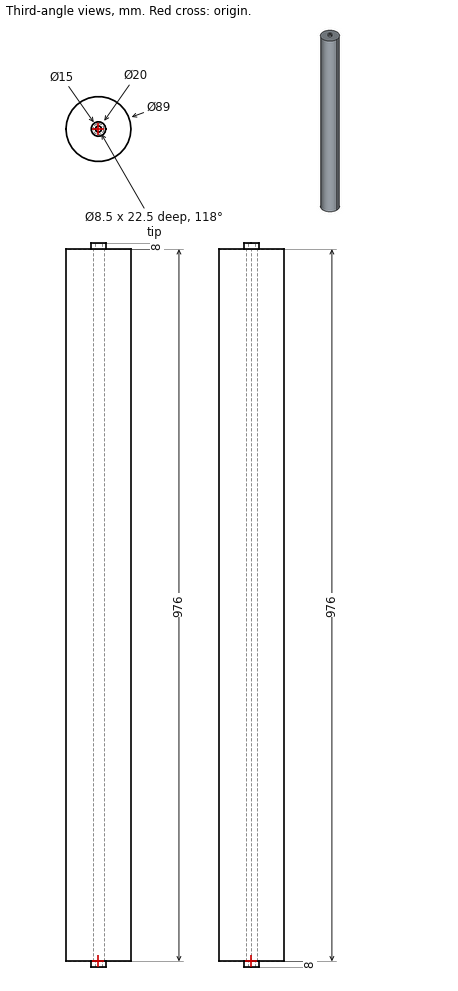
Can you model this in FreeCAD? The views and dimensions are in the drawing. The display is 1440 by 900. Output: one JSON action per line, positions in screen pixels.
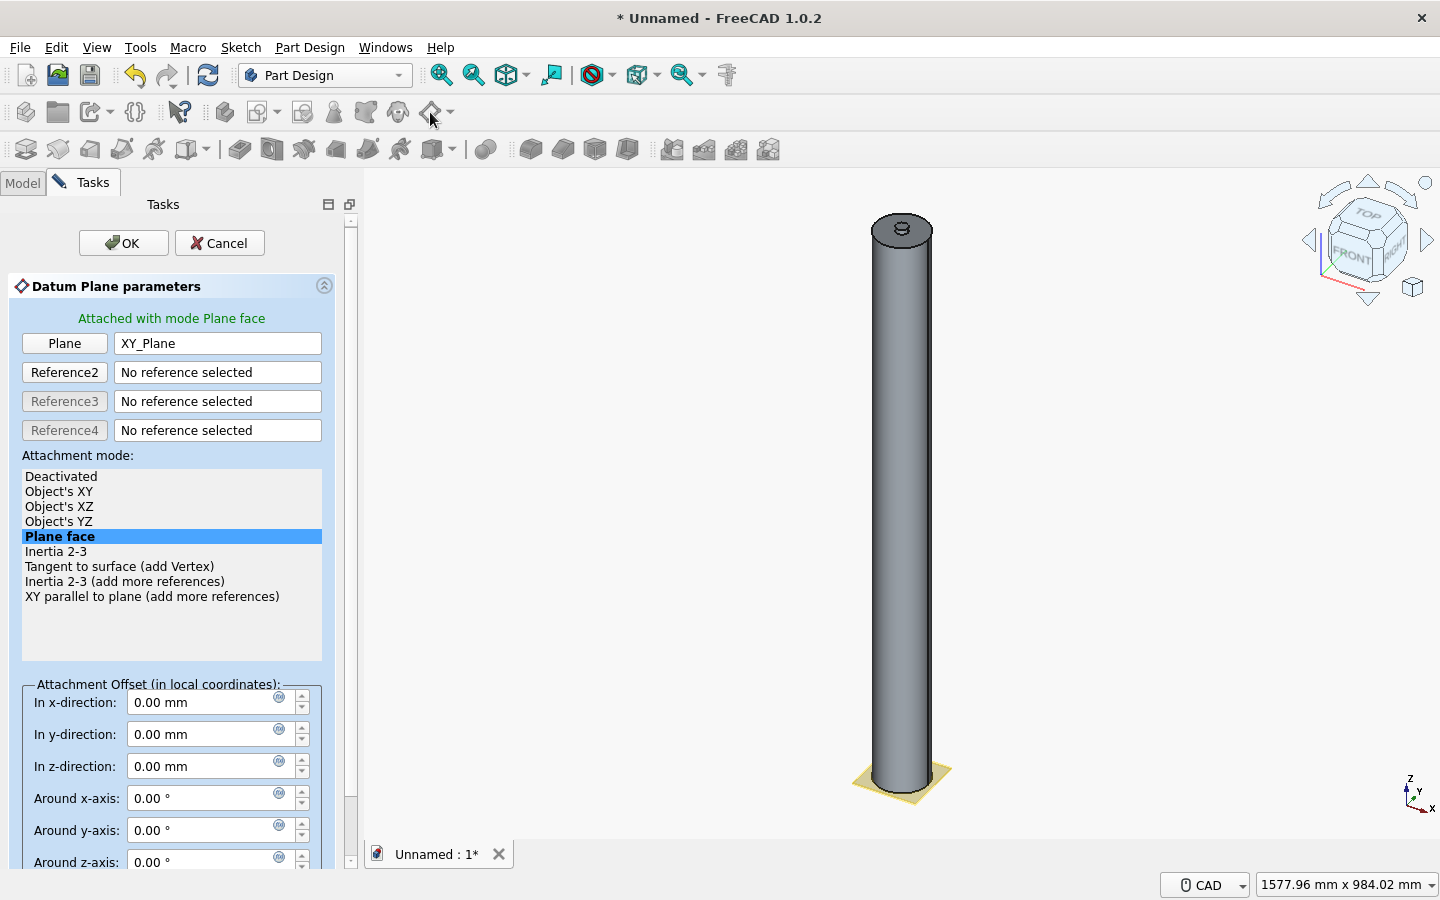
{"action": "triple_click", "coordinate": [210, 766]}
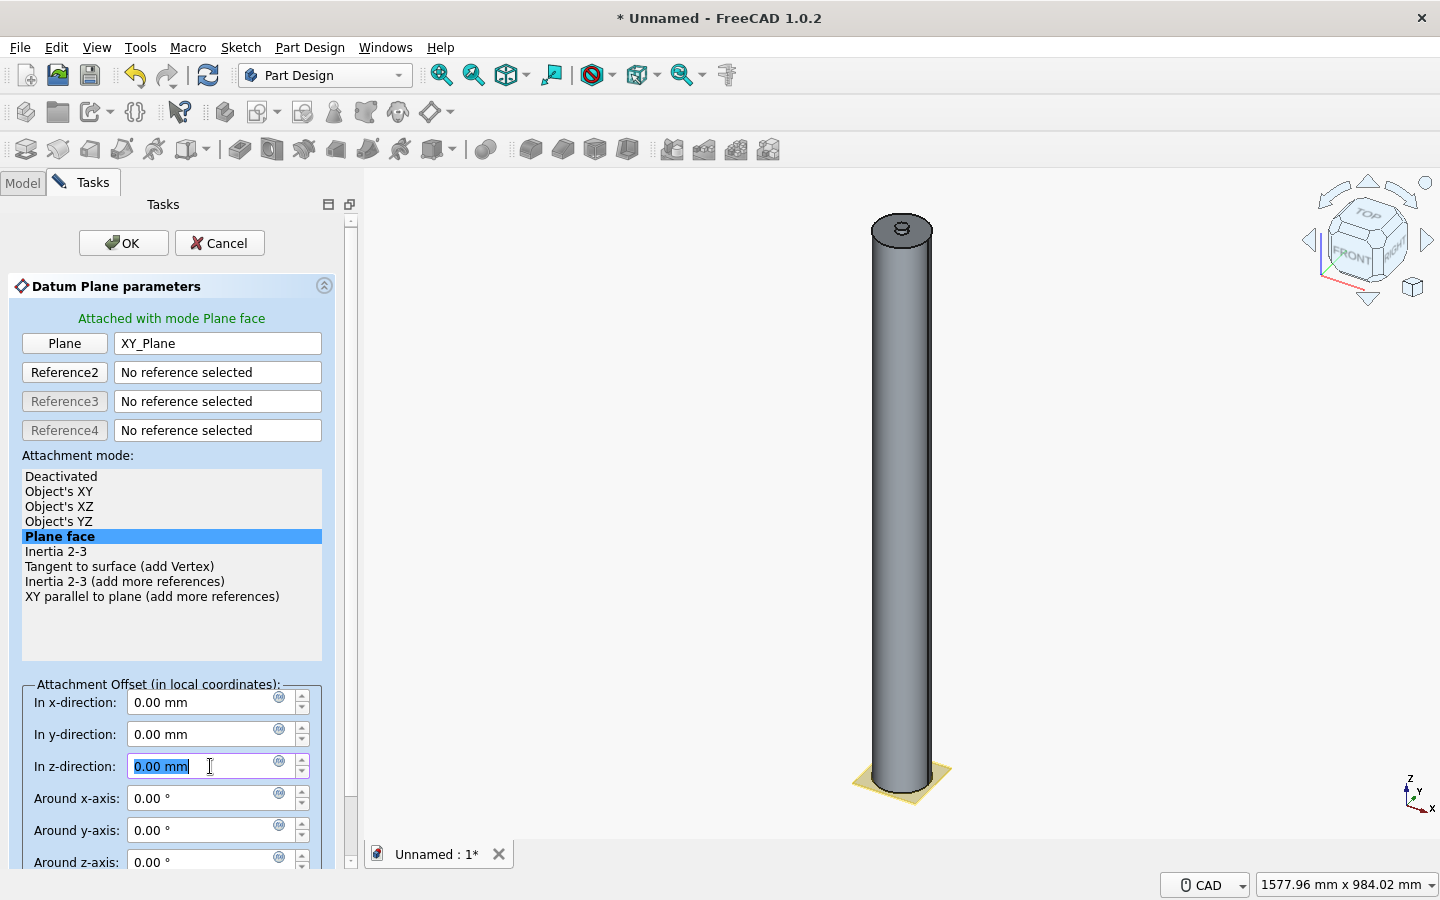
{"action": "type", "text": "-8"}
{"action": "key", "text": "Tab"}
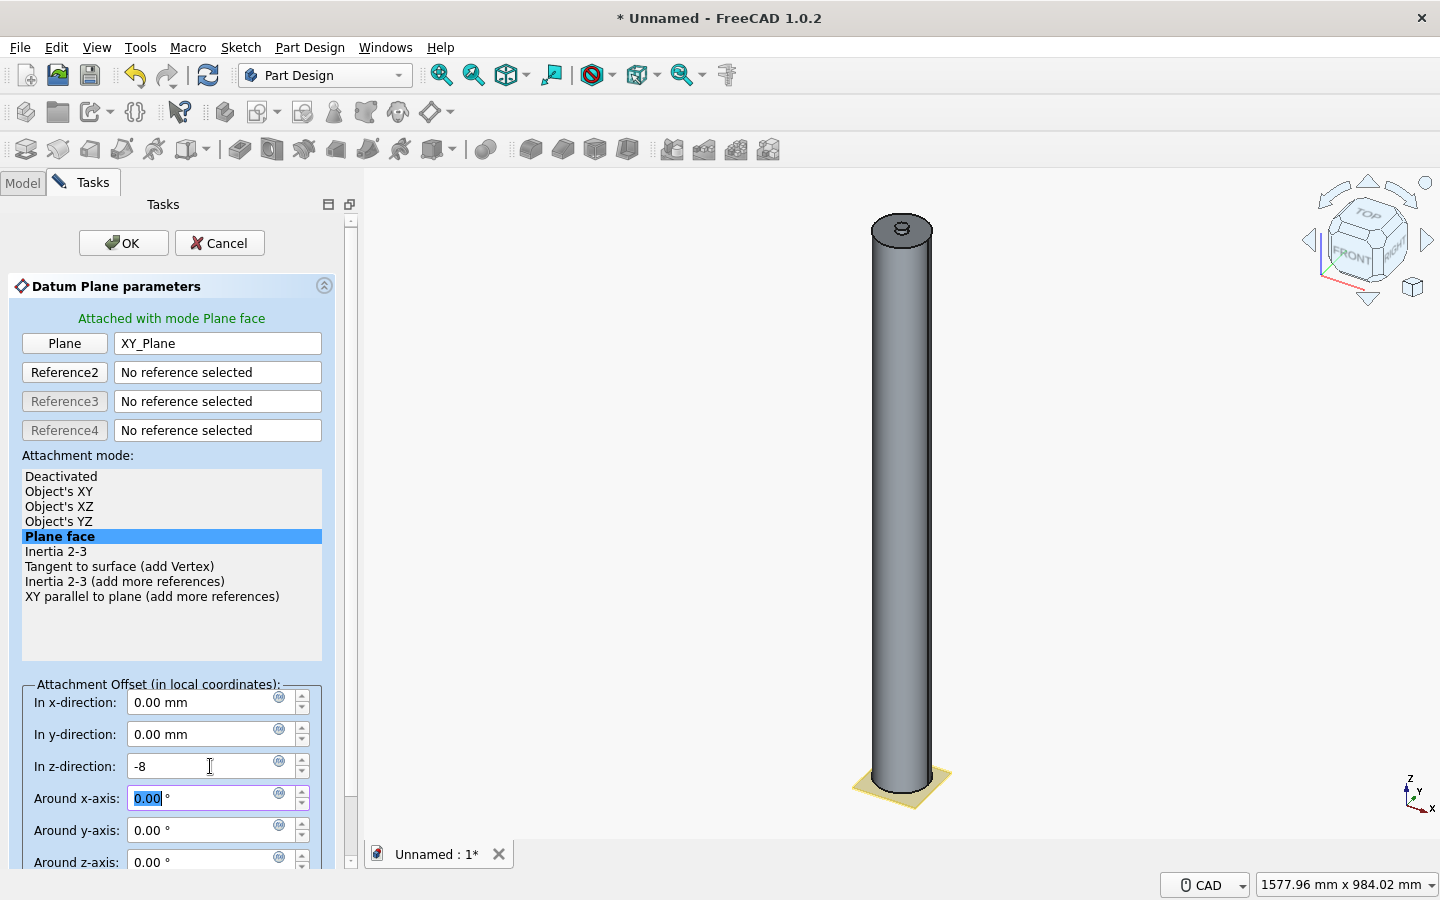
{"action": "left_click", "coordinate": [124, 243]}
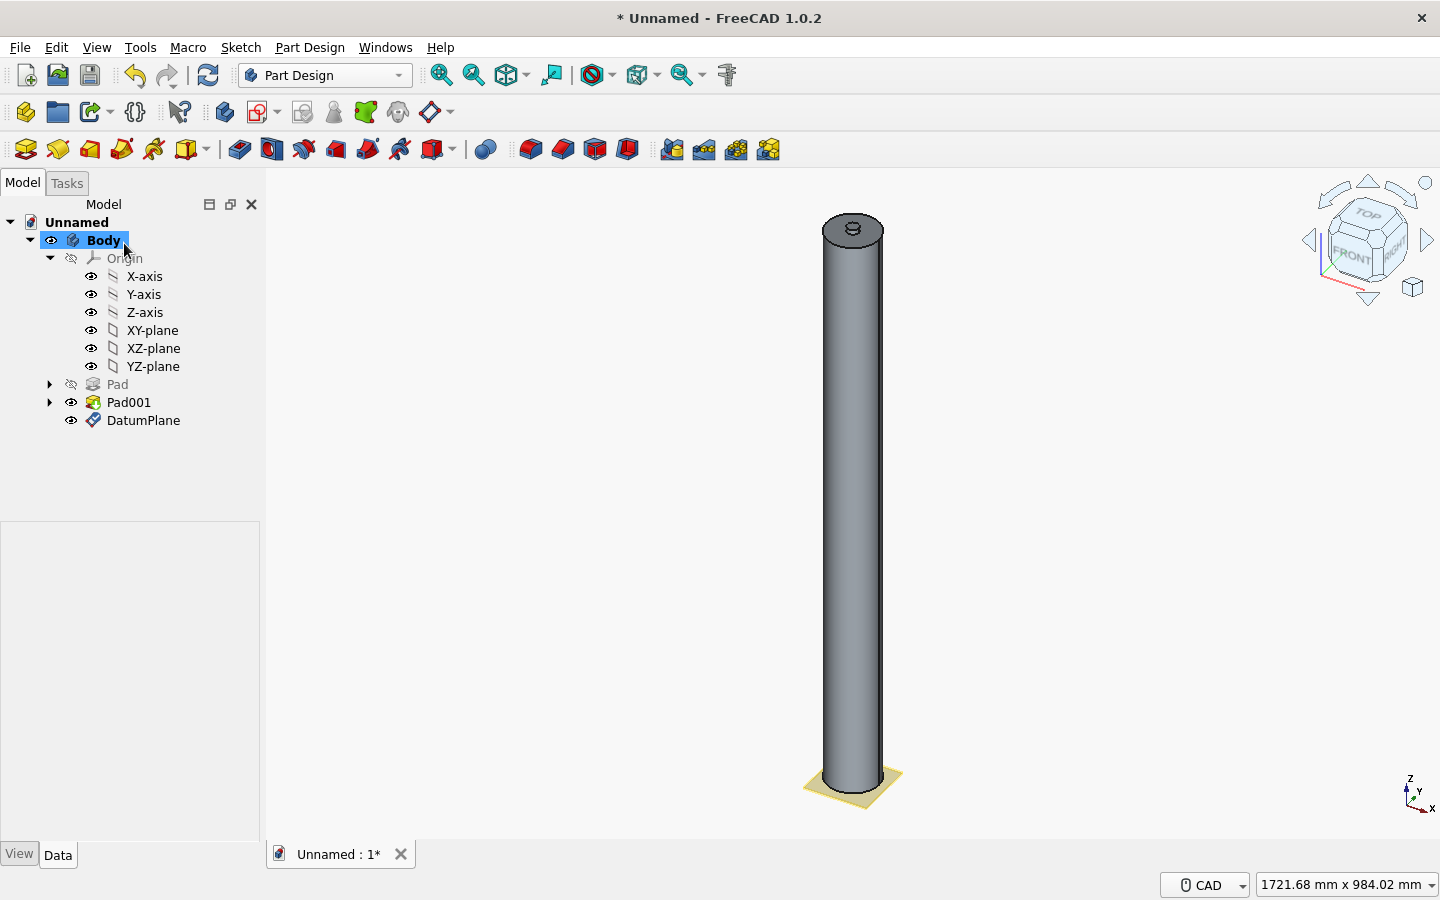
{"action": "left_click", "coordinate": [116, 420]}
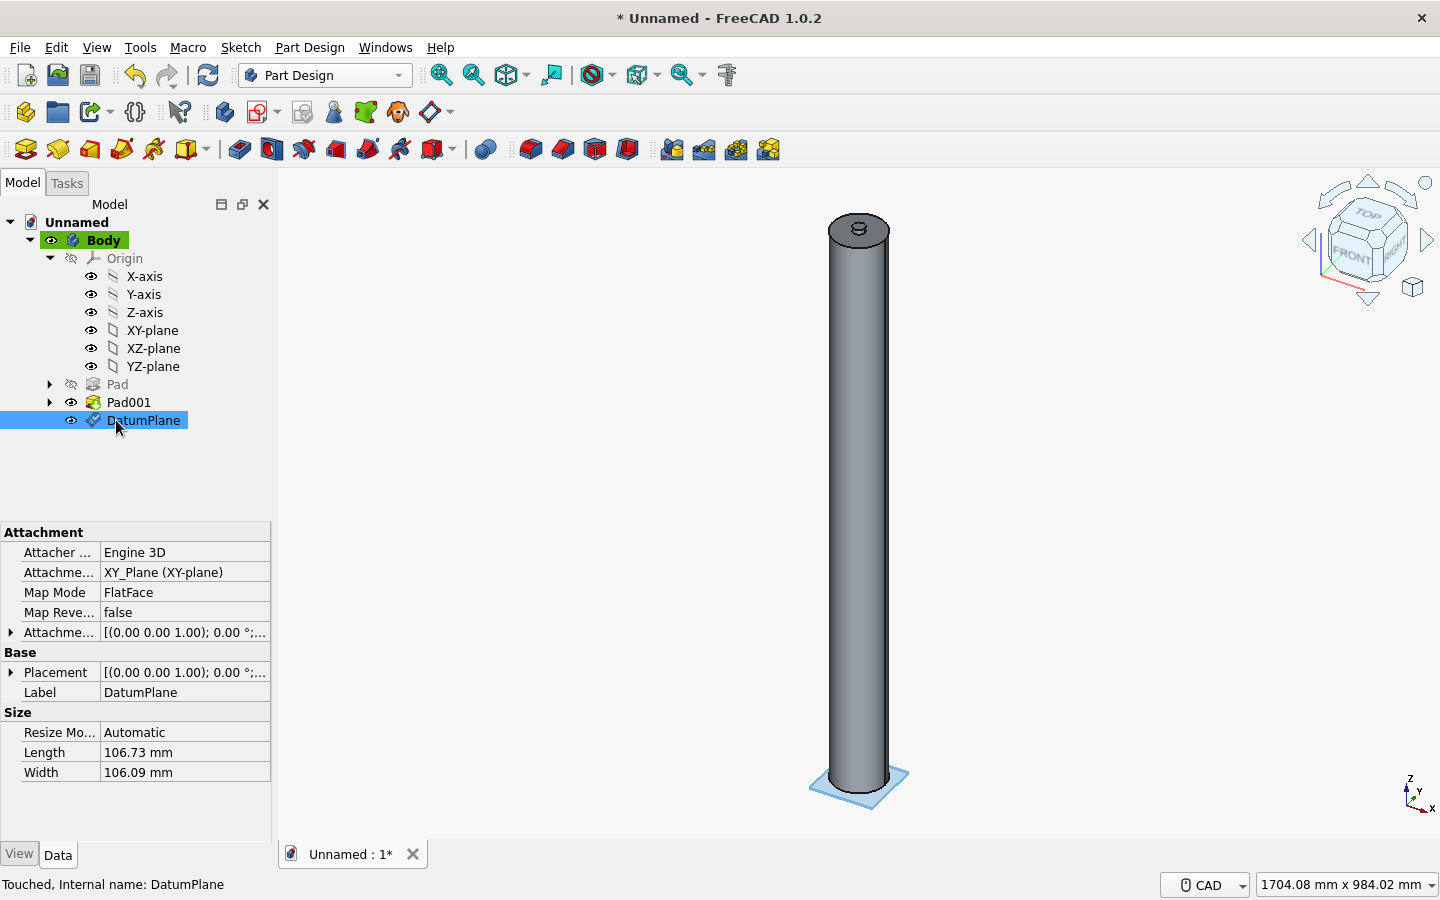
{"action": "left_click", "coordinate": [258, 112]}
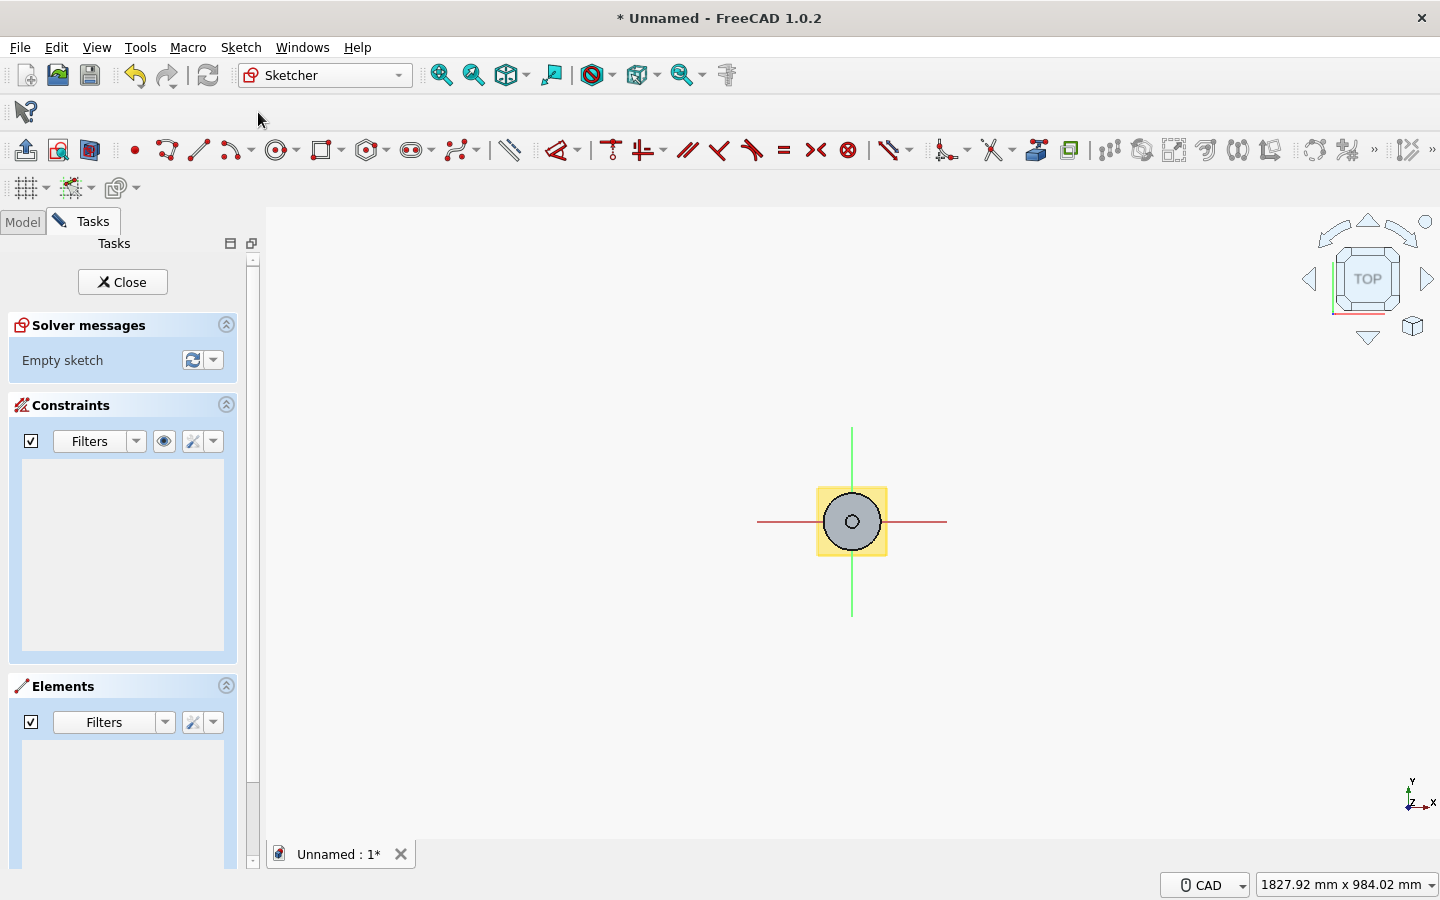
{"action": "left_click", "coordinate": [90, 150]}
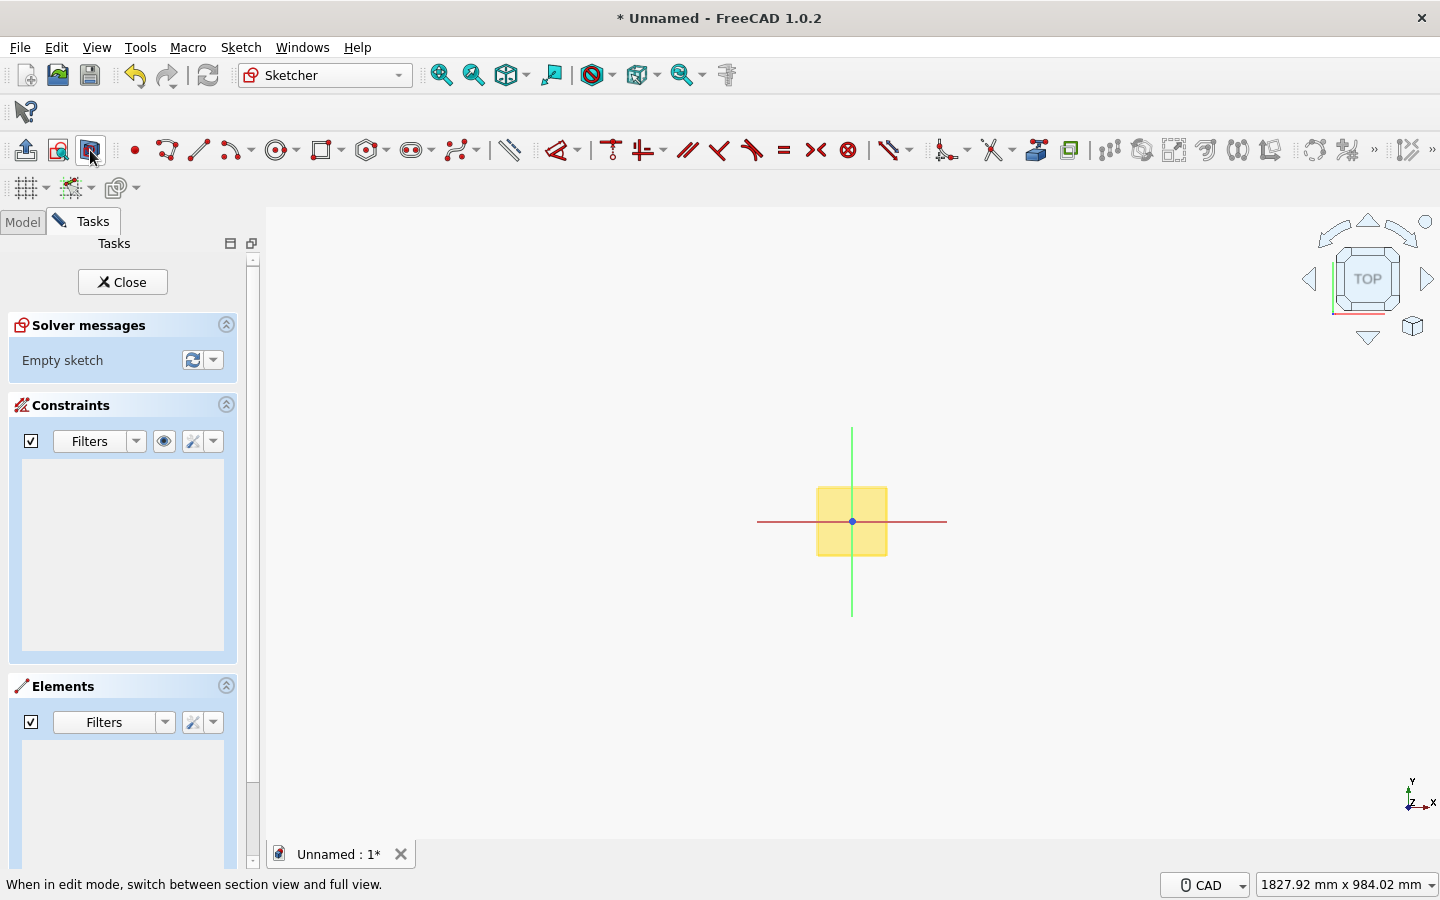
{"action": "scroll", "coordinate": [856, 522], "scroll_direction": "up", "scroll_amount": 15}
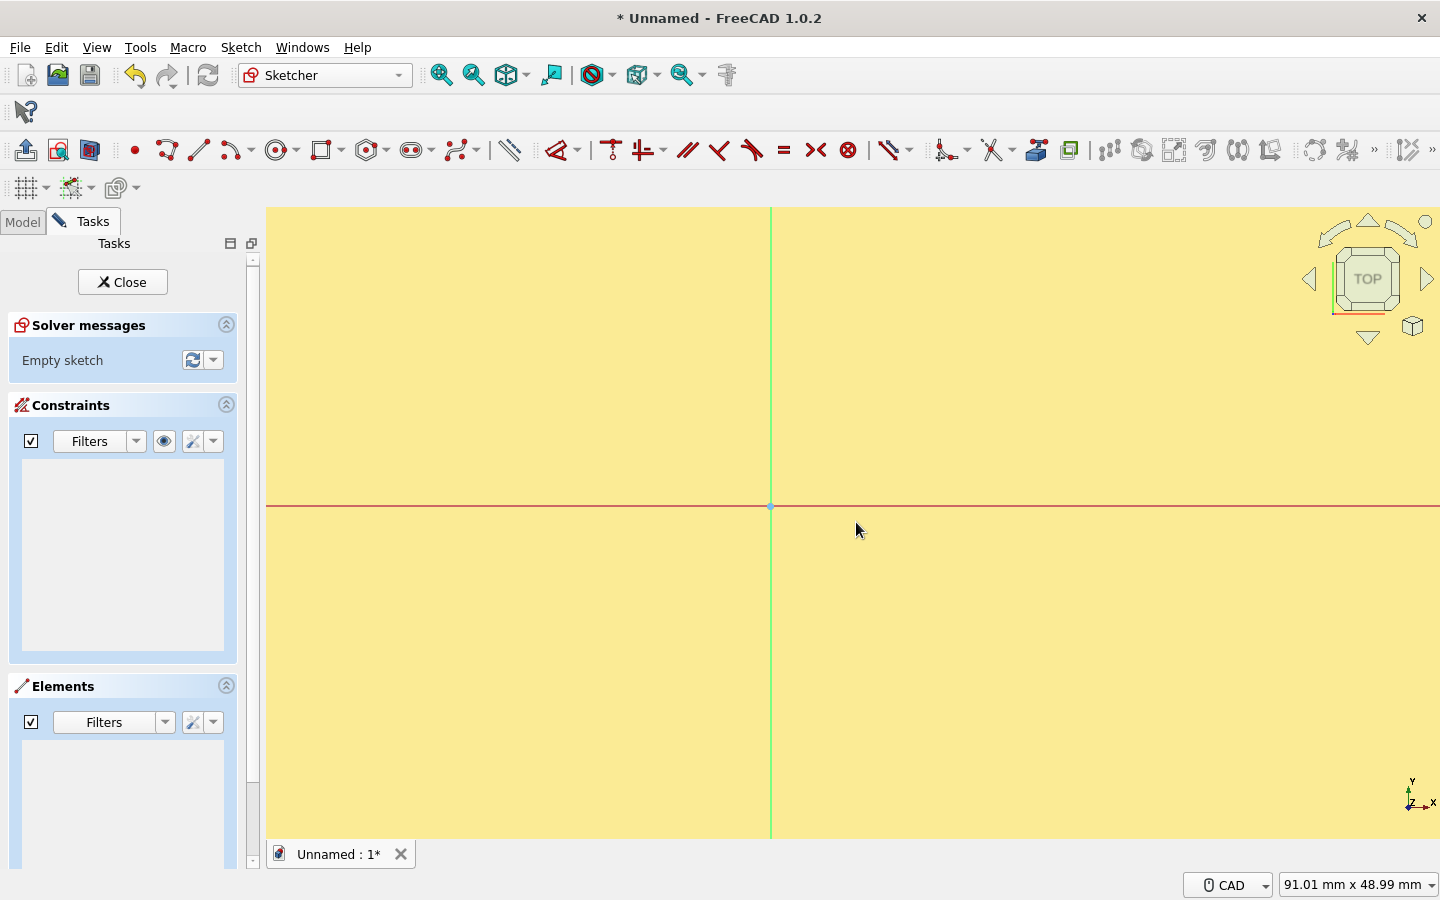
{"action": "scroll", "coordinate": [743, 472], "scroll_direction": "up", "scroll_amount": 2}